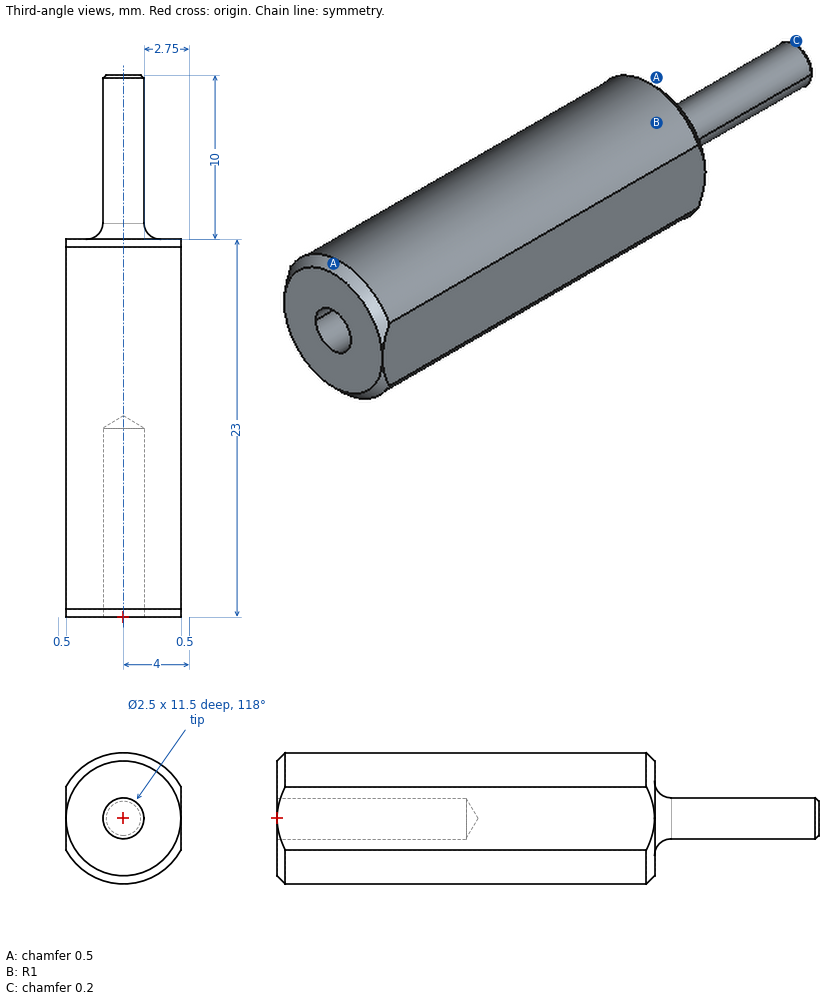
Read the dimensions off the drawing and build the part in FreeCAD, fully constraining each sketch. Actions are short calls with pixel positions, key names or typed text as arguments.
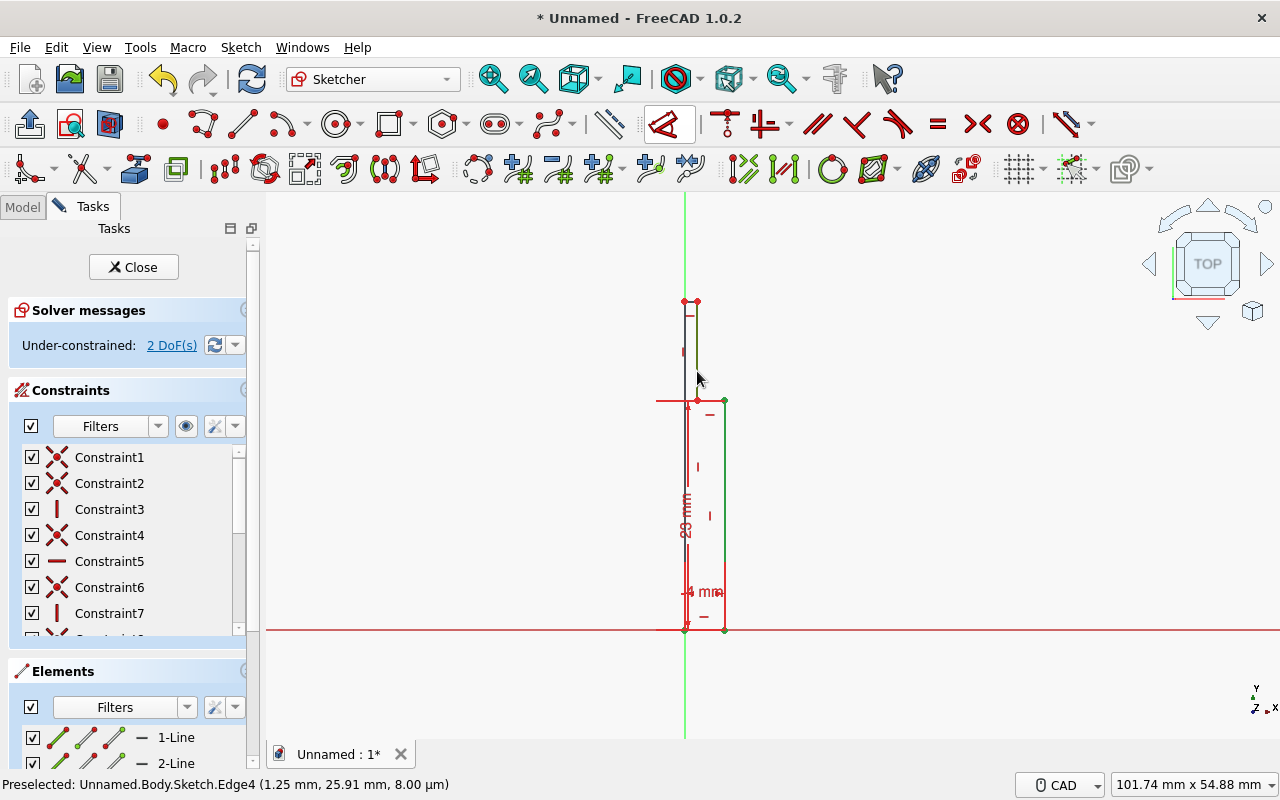
key(i)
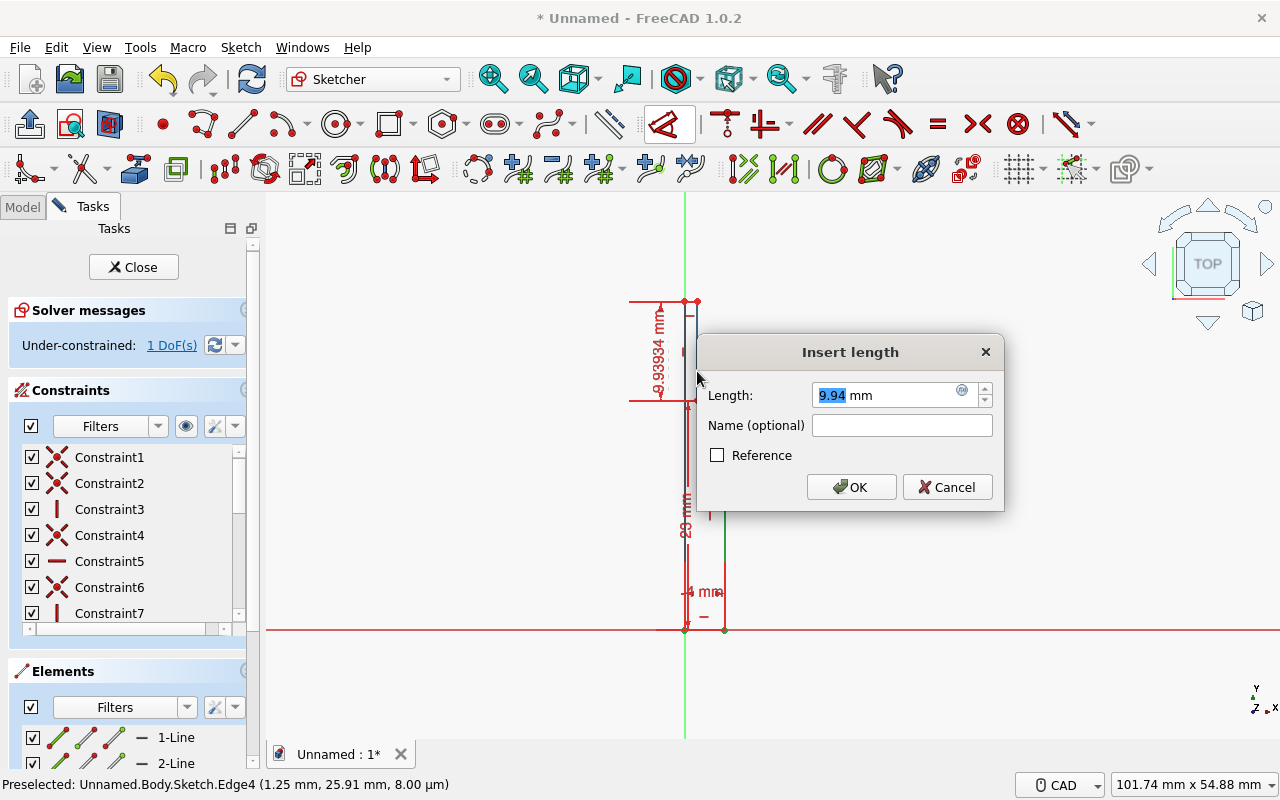
text(10)
key(Return)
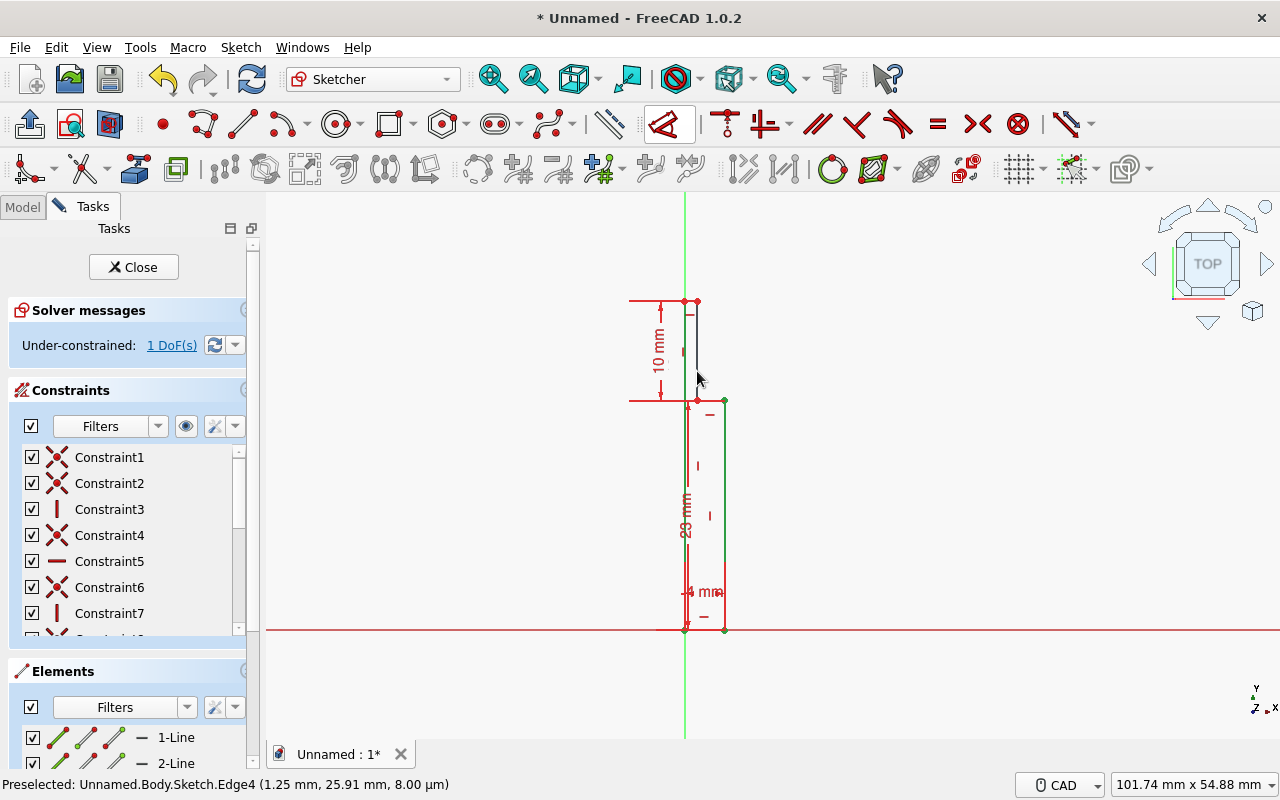
scroll(714, 401, up, 2)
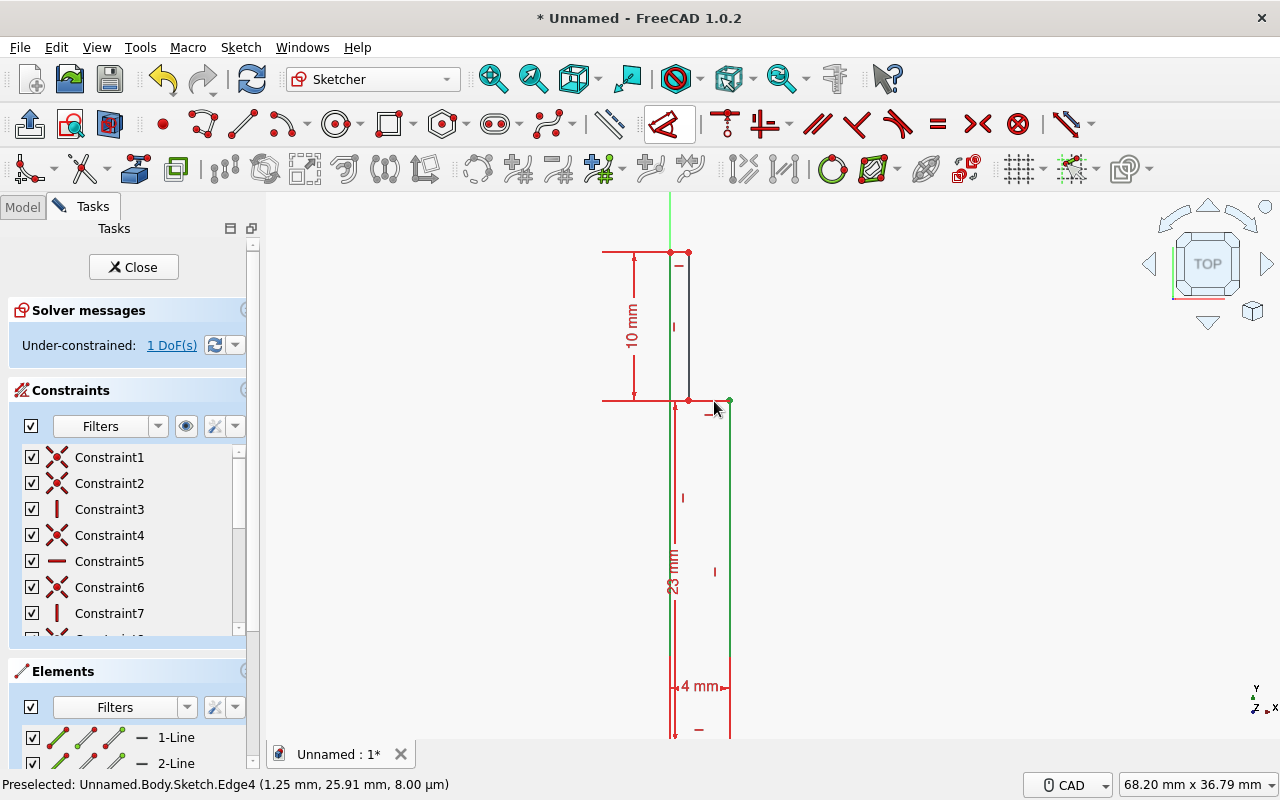
click(713, 401)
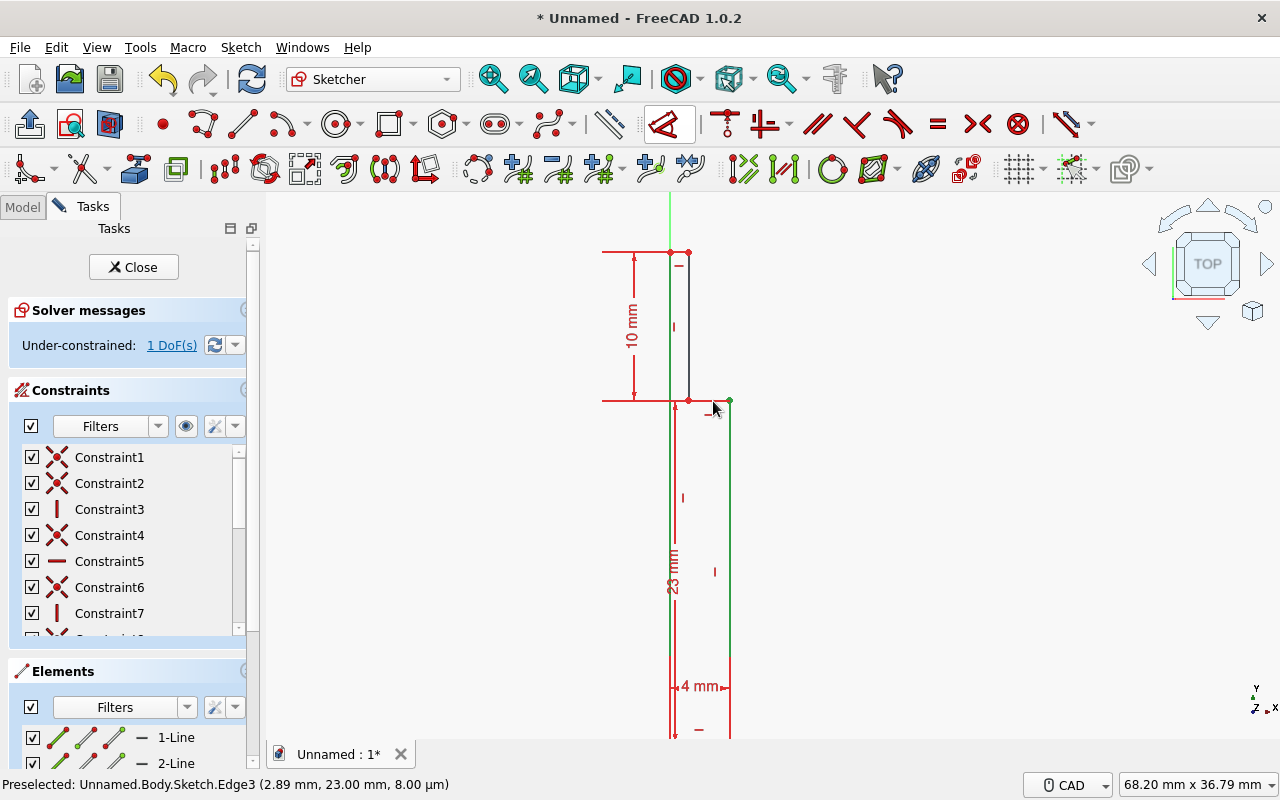
key(l)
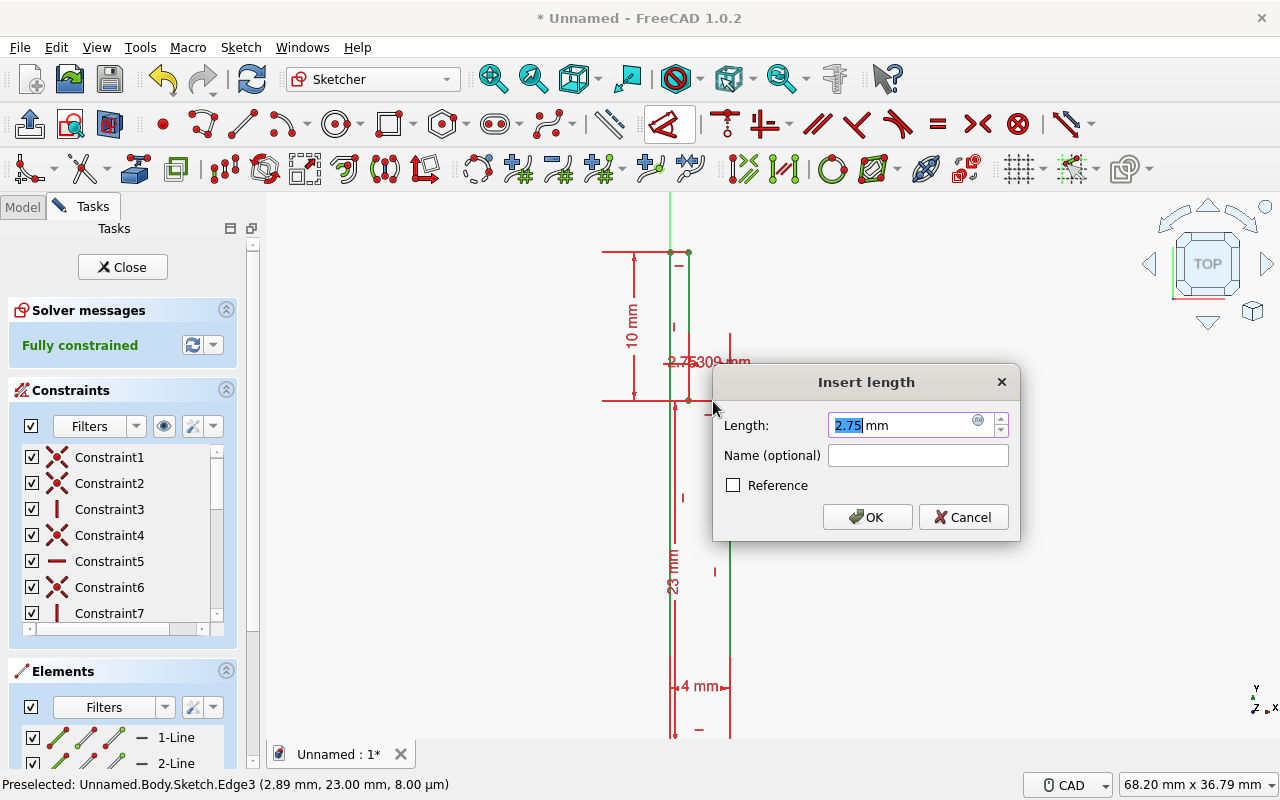
text(2.75)
key(Return)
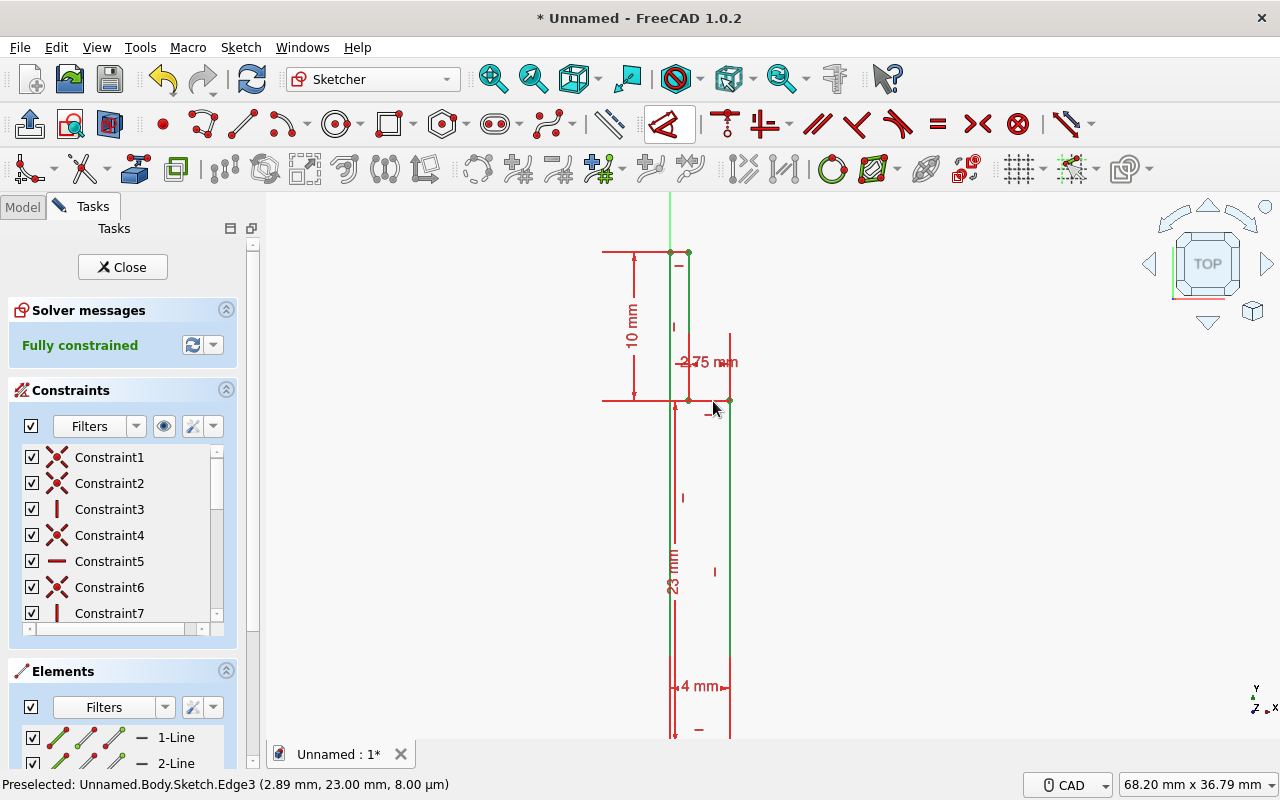
click(123, 267)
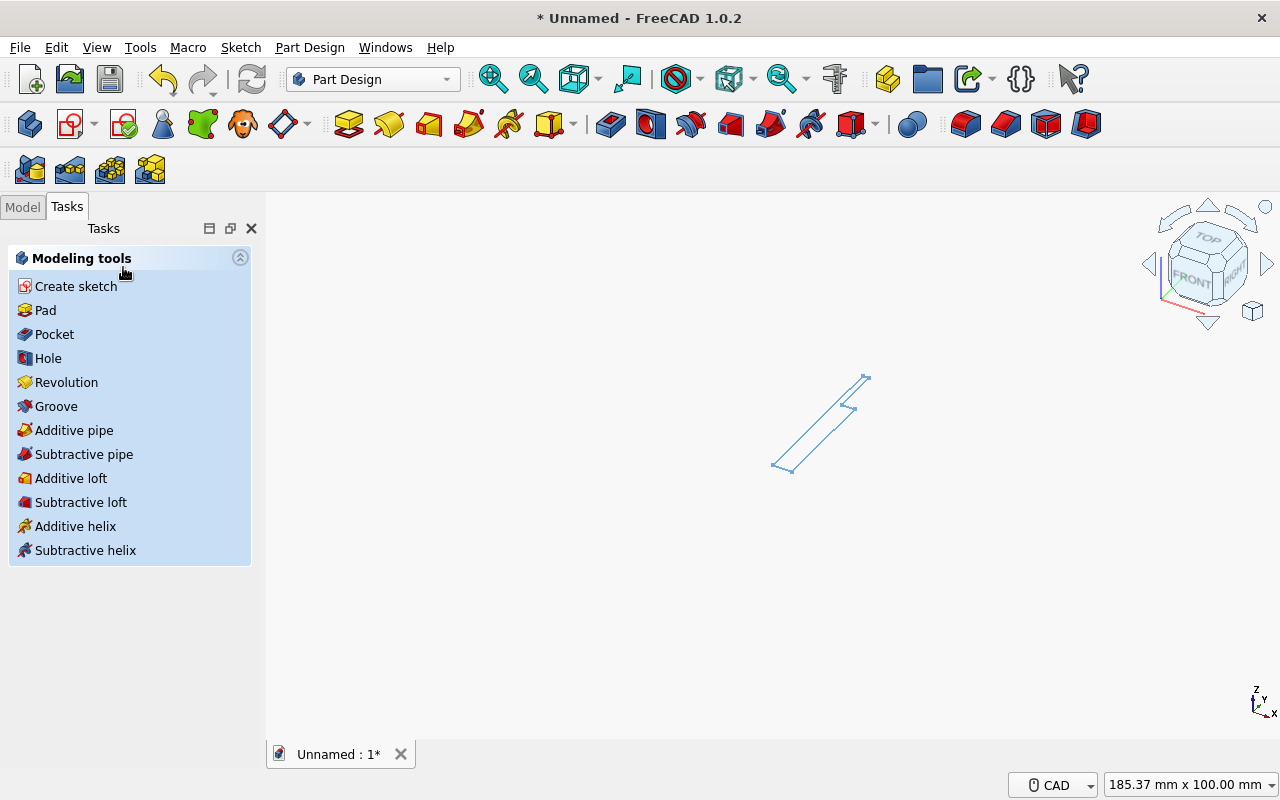
click(390, 124)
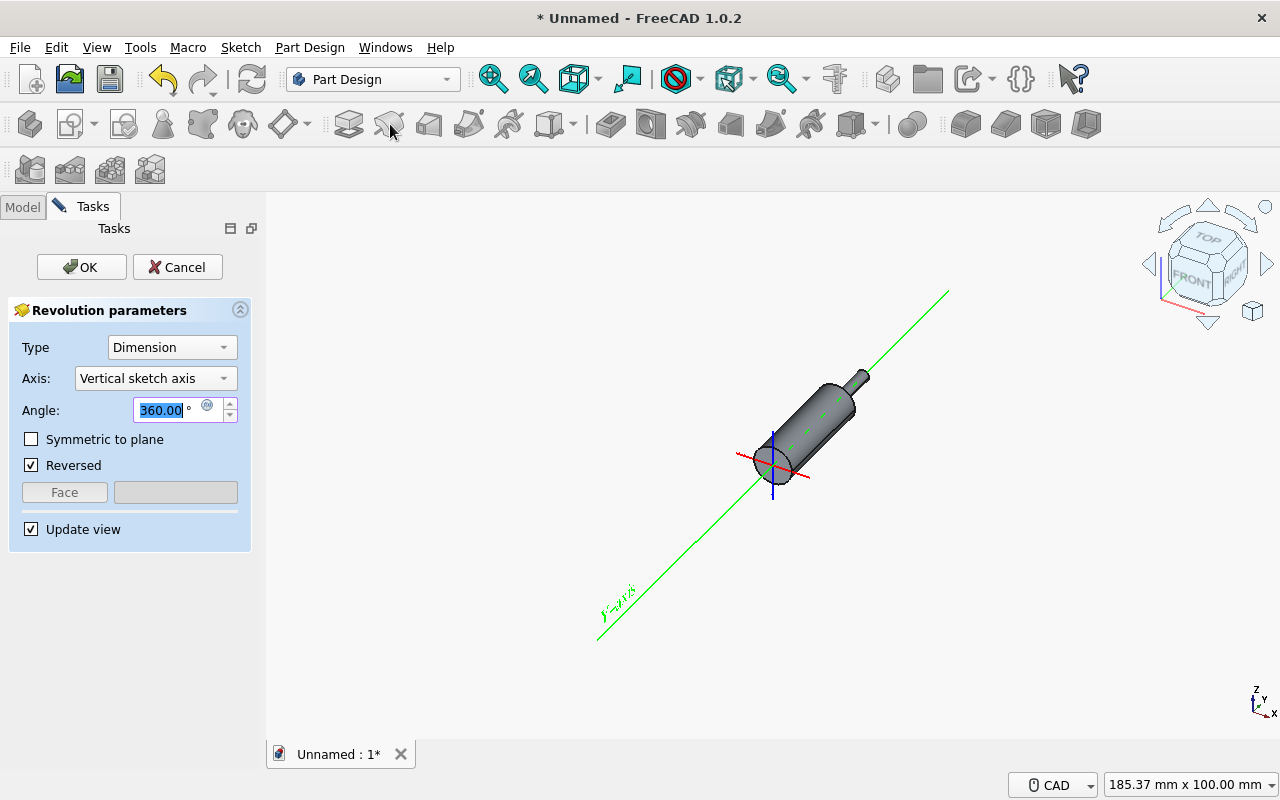
click(82, 267)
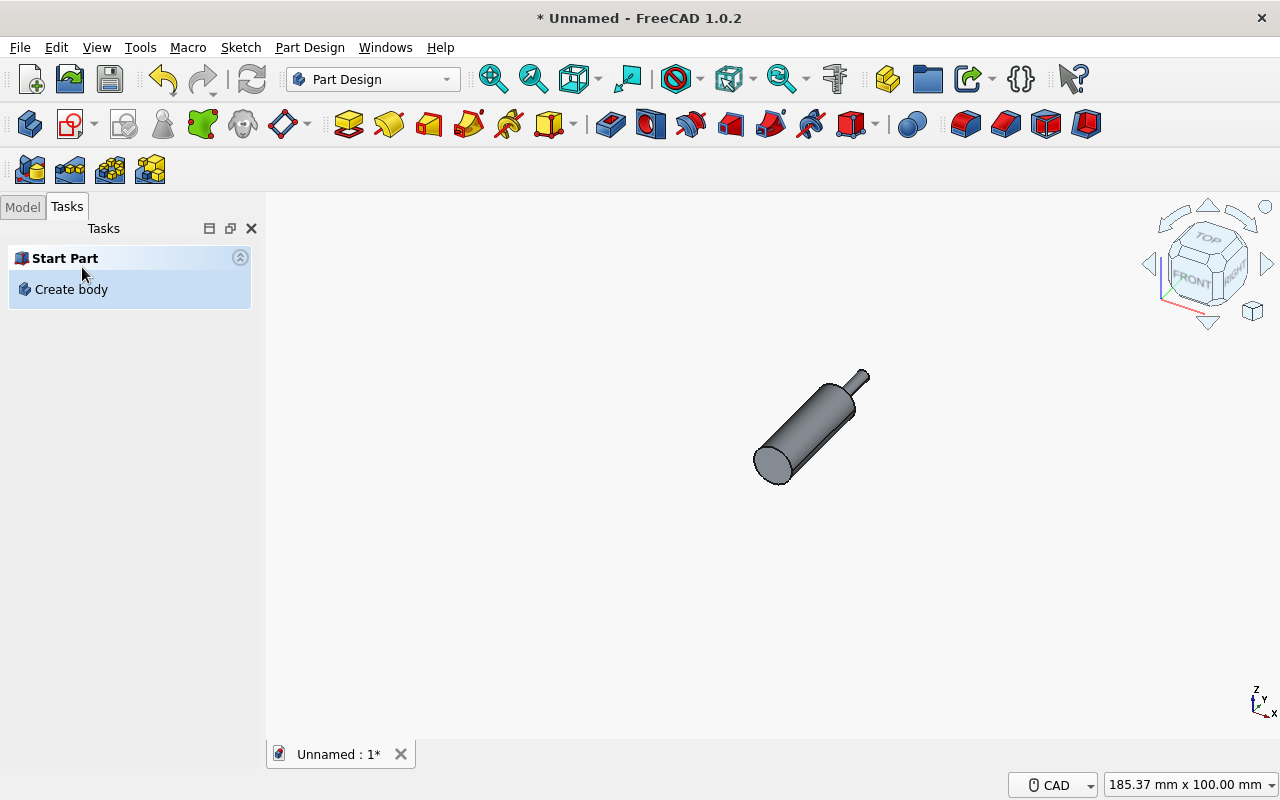
key(v)
key(f)